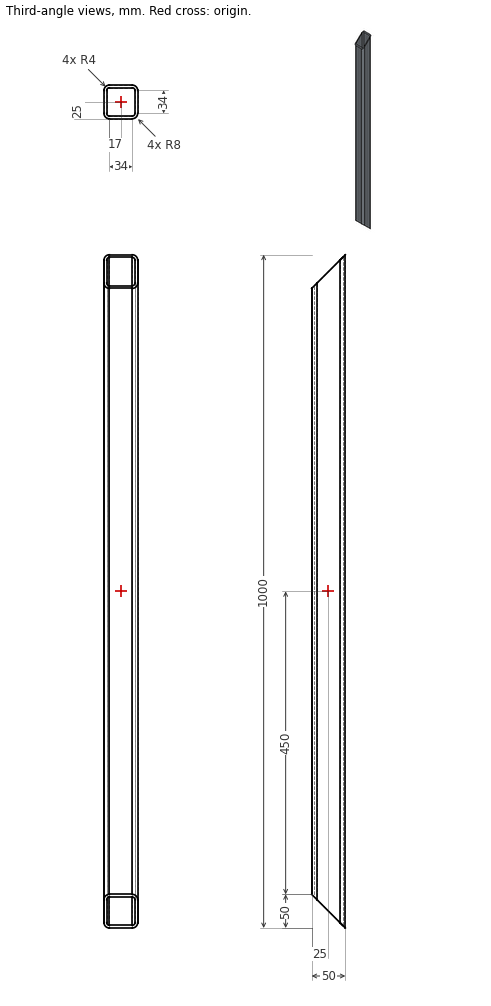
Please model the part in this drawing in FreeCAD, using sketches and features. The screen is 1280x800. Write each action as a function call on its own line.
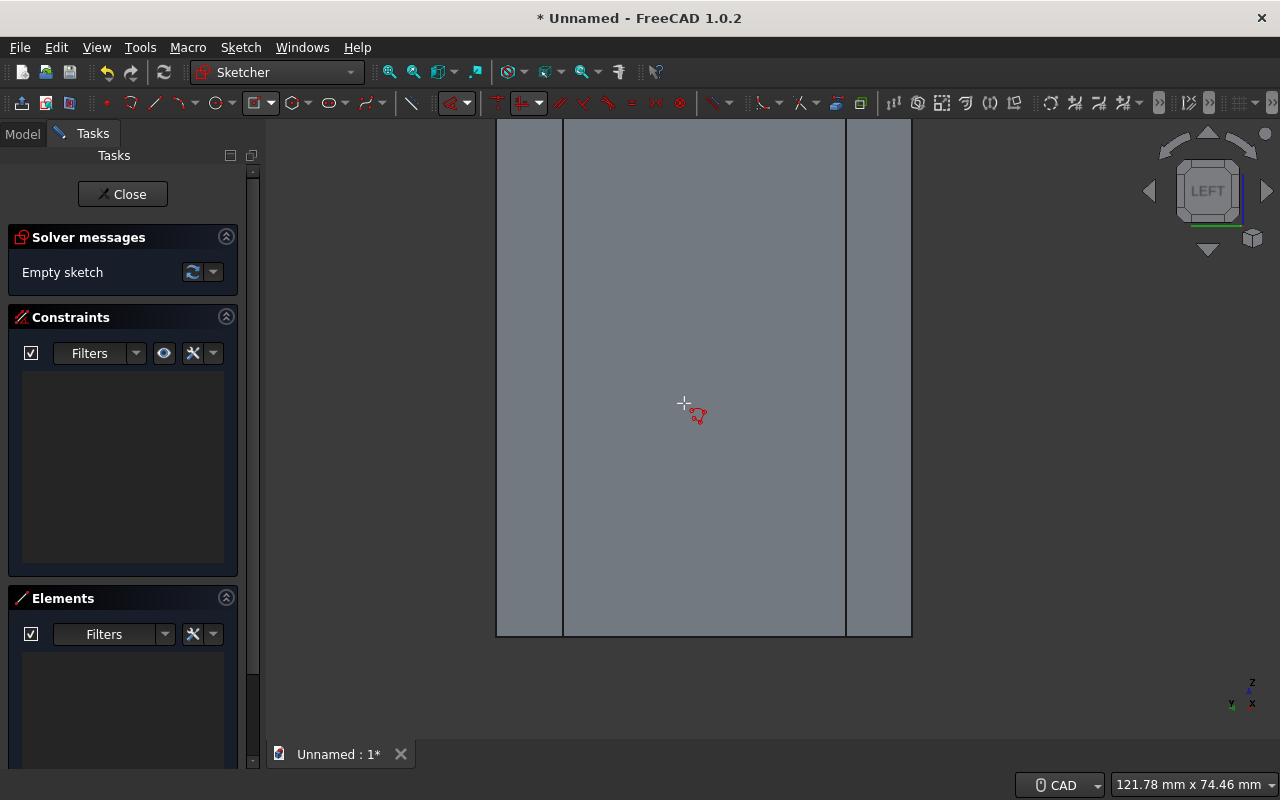
click(912, 220)
click(496, 637)
click(912, 637)
click(912, 221)
key(Escape)
key(Escape)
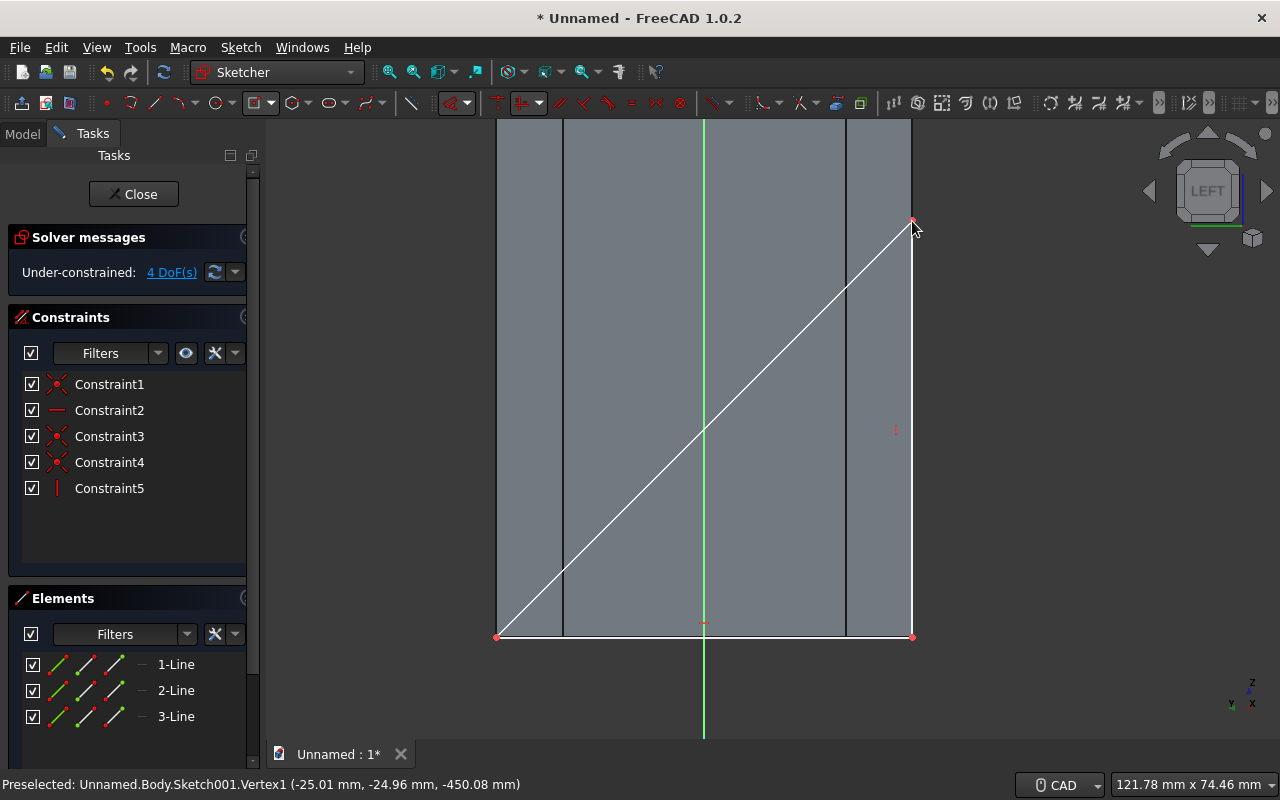
key(d)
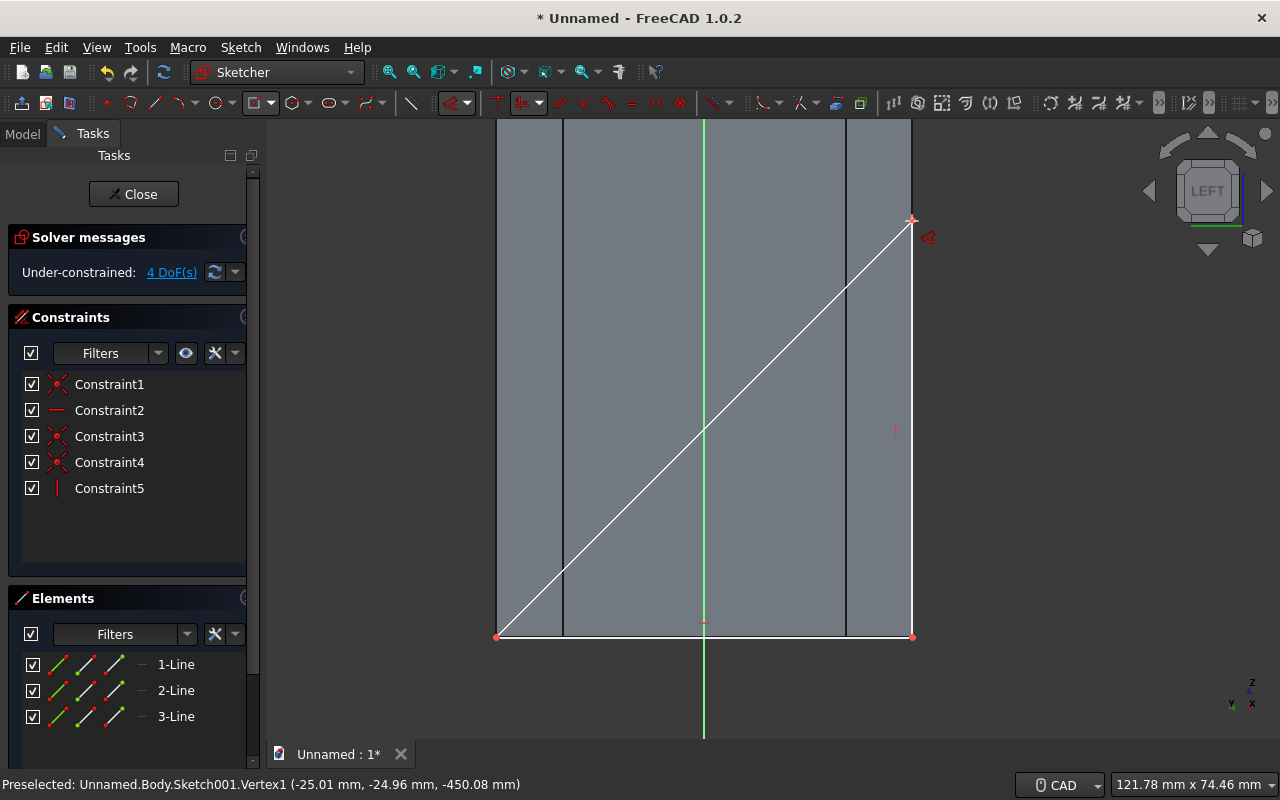
click(621, 638)
click(608, 672)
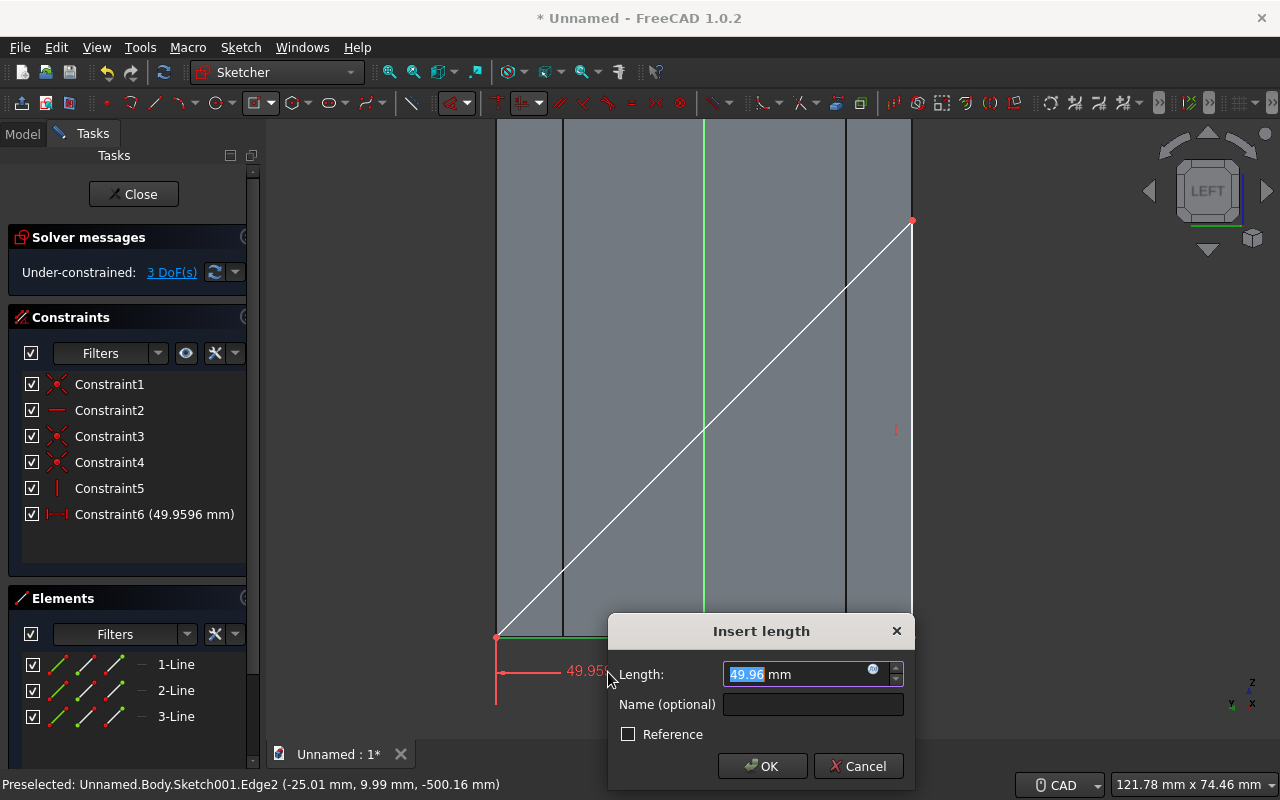
text(50)
key(Return)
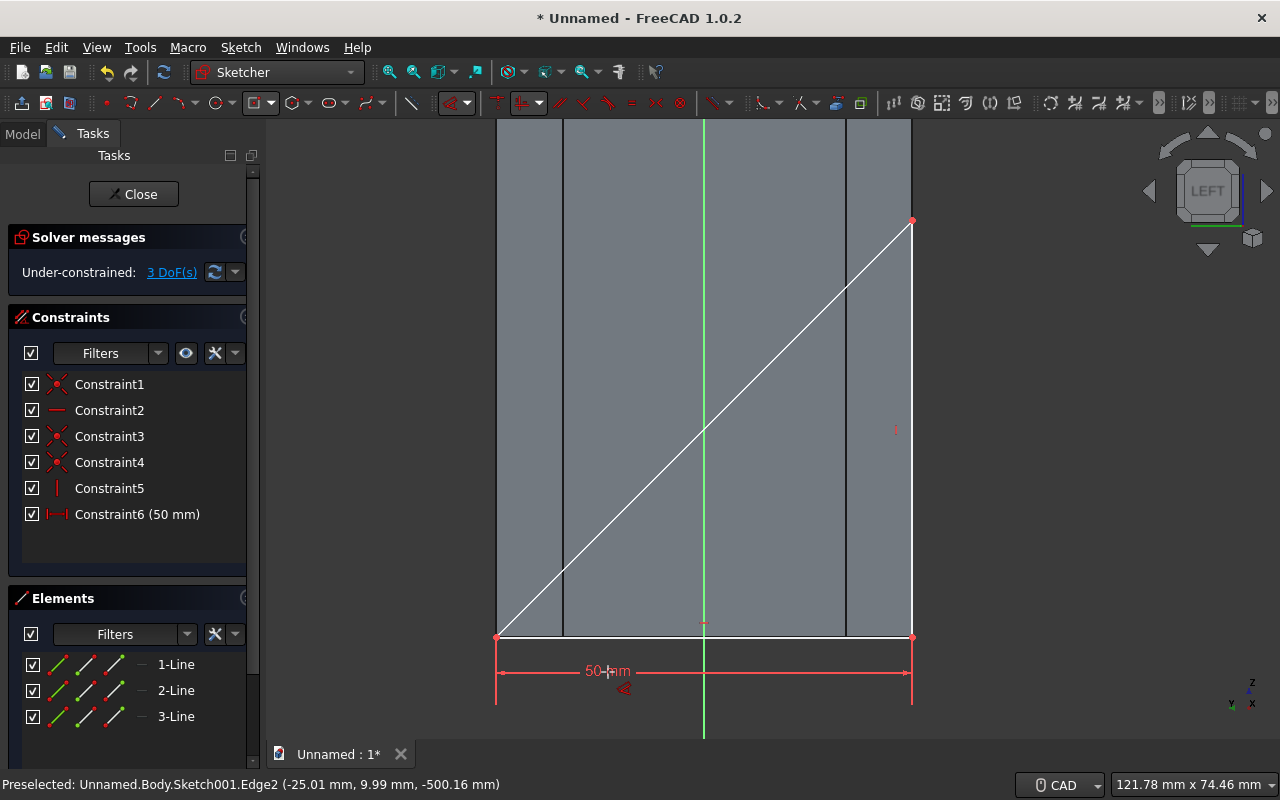
click(912, 513)
click(946, 430)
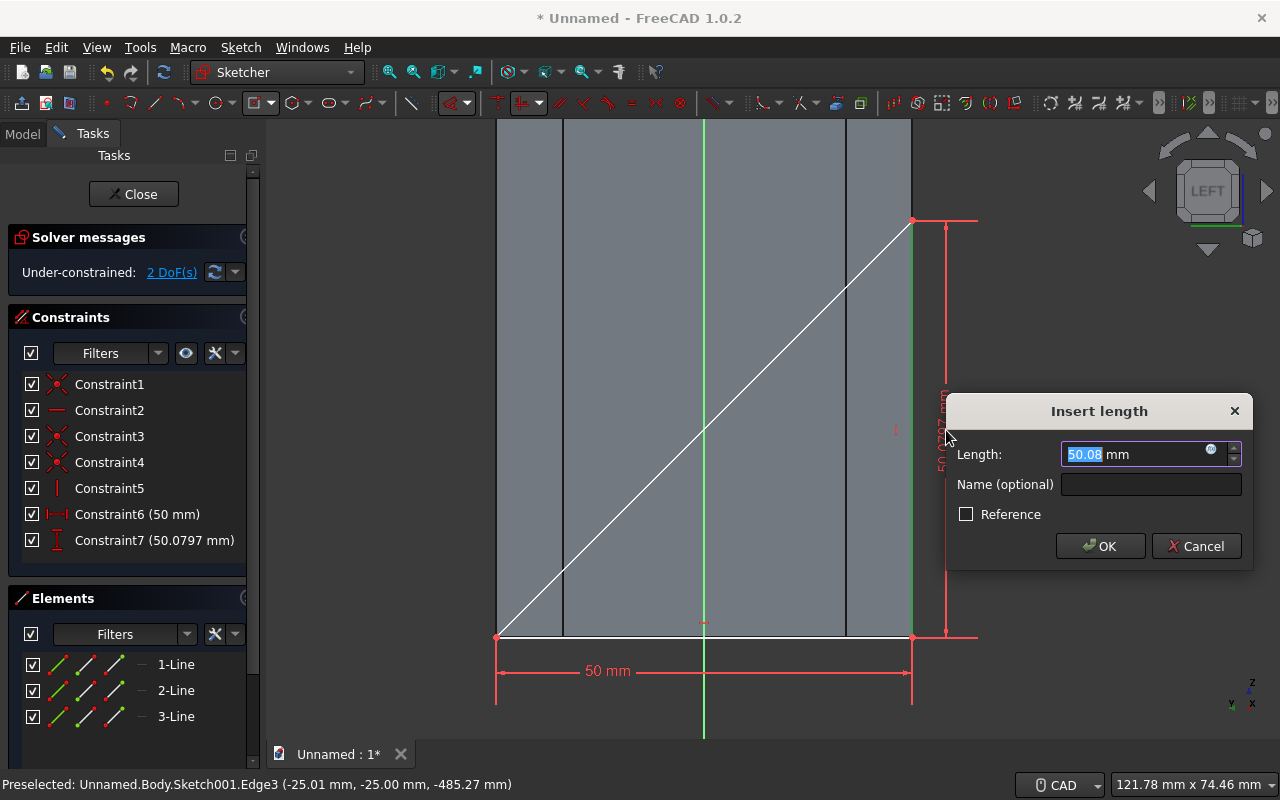
text(50)
key(Return)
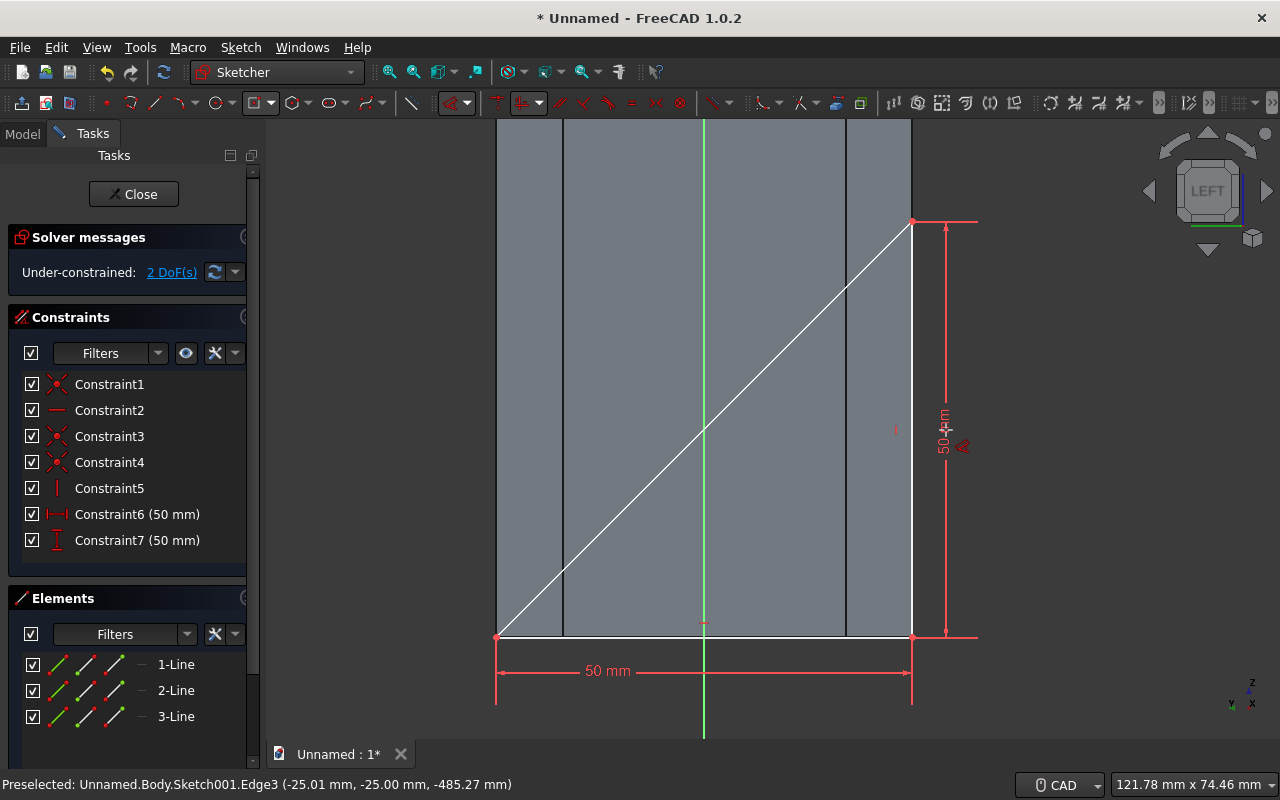
click(912, 222)
click(808, 256)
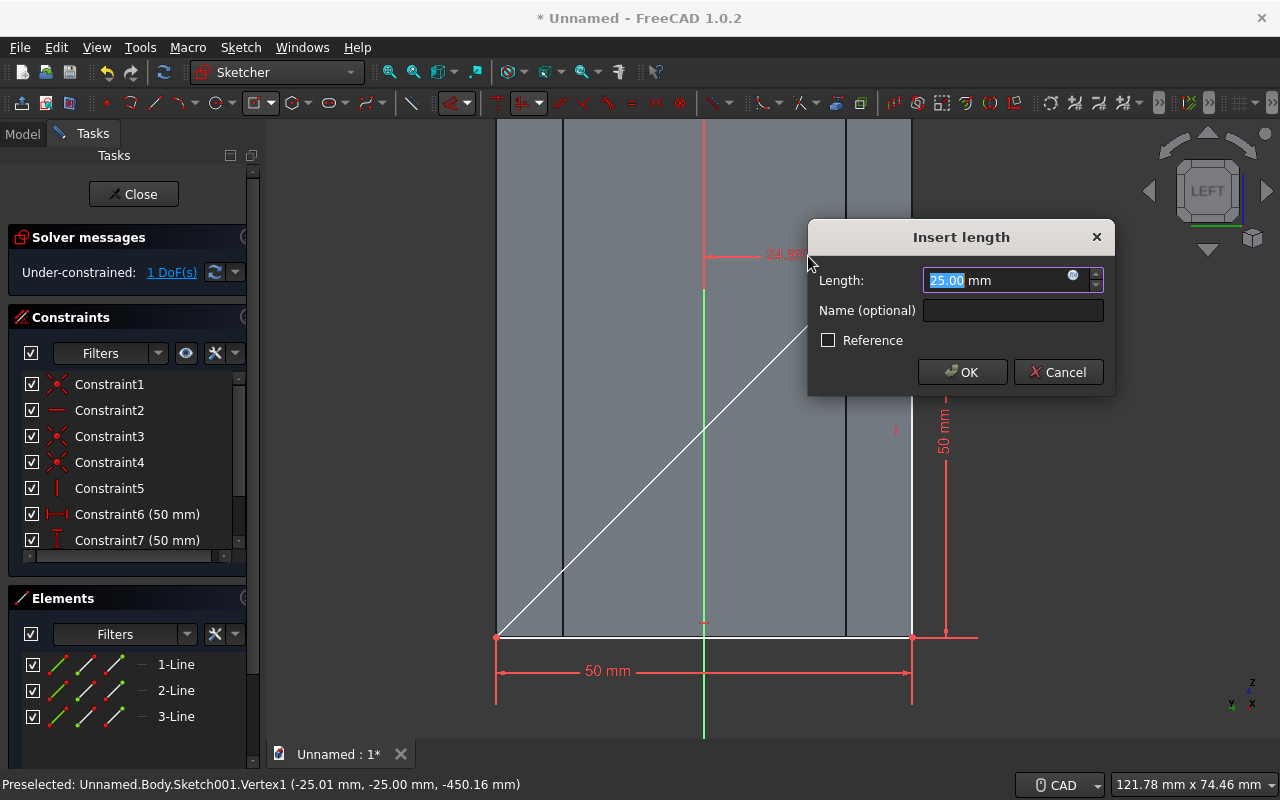
text(25)
key(Return)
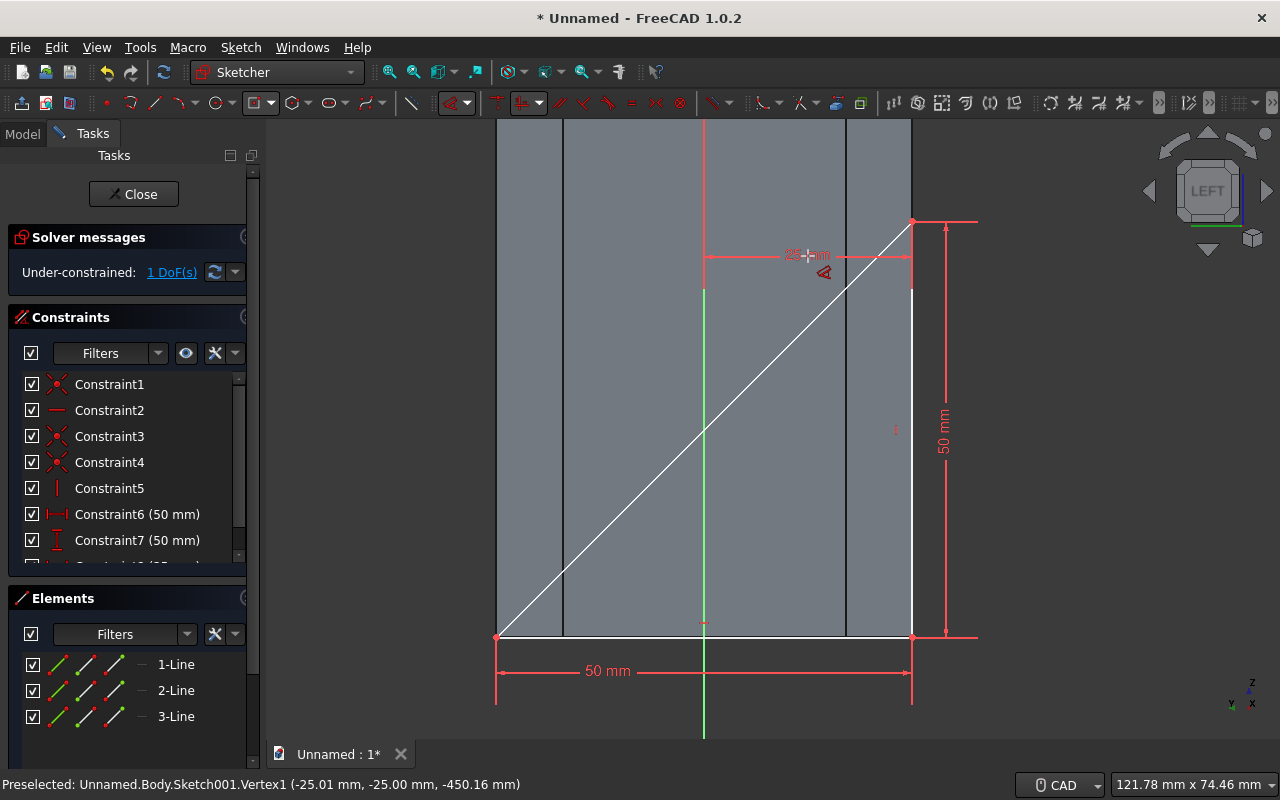
click(912, 222)
click(946, 184)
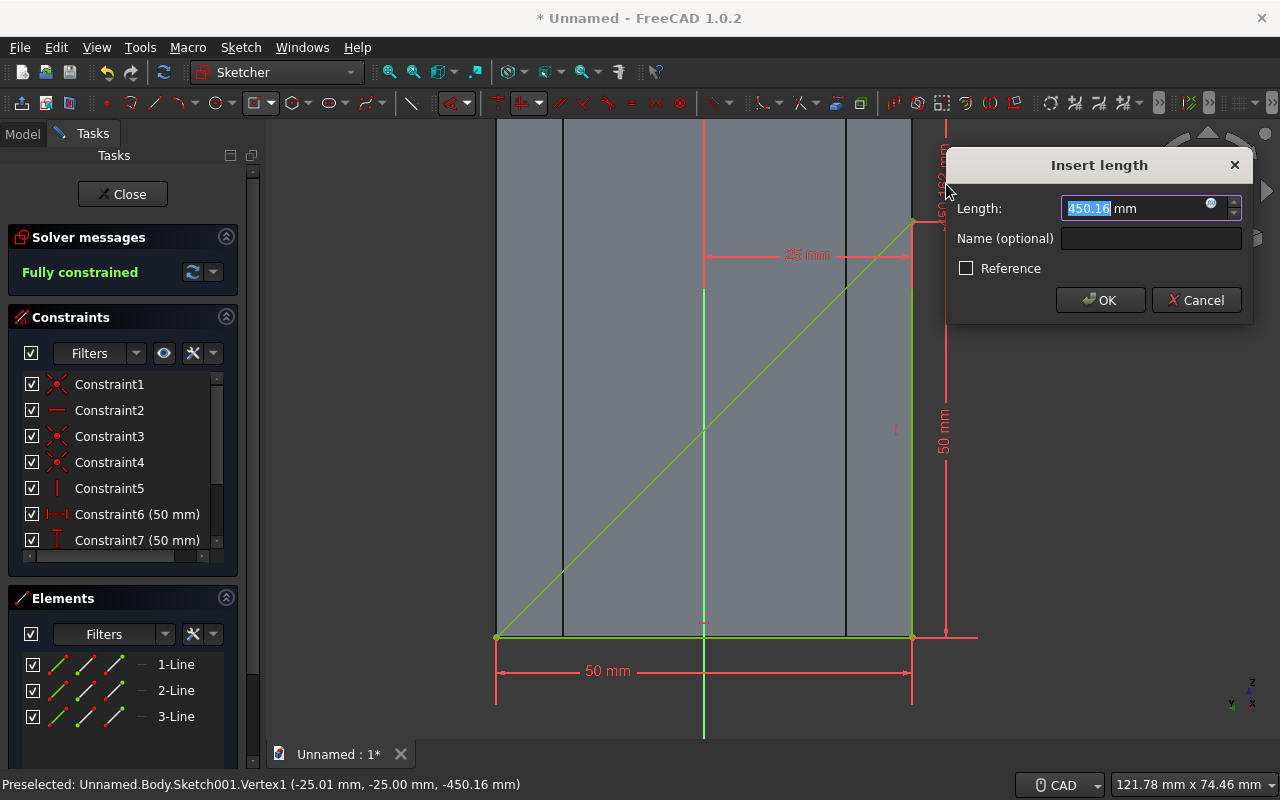
text(450)
key(Return)
key(Escape)